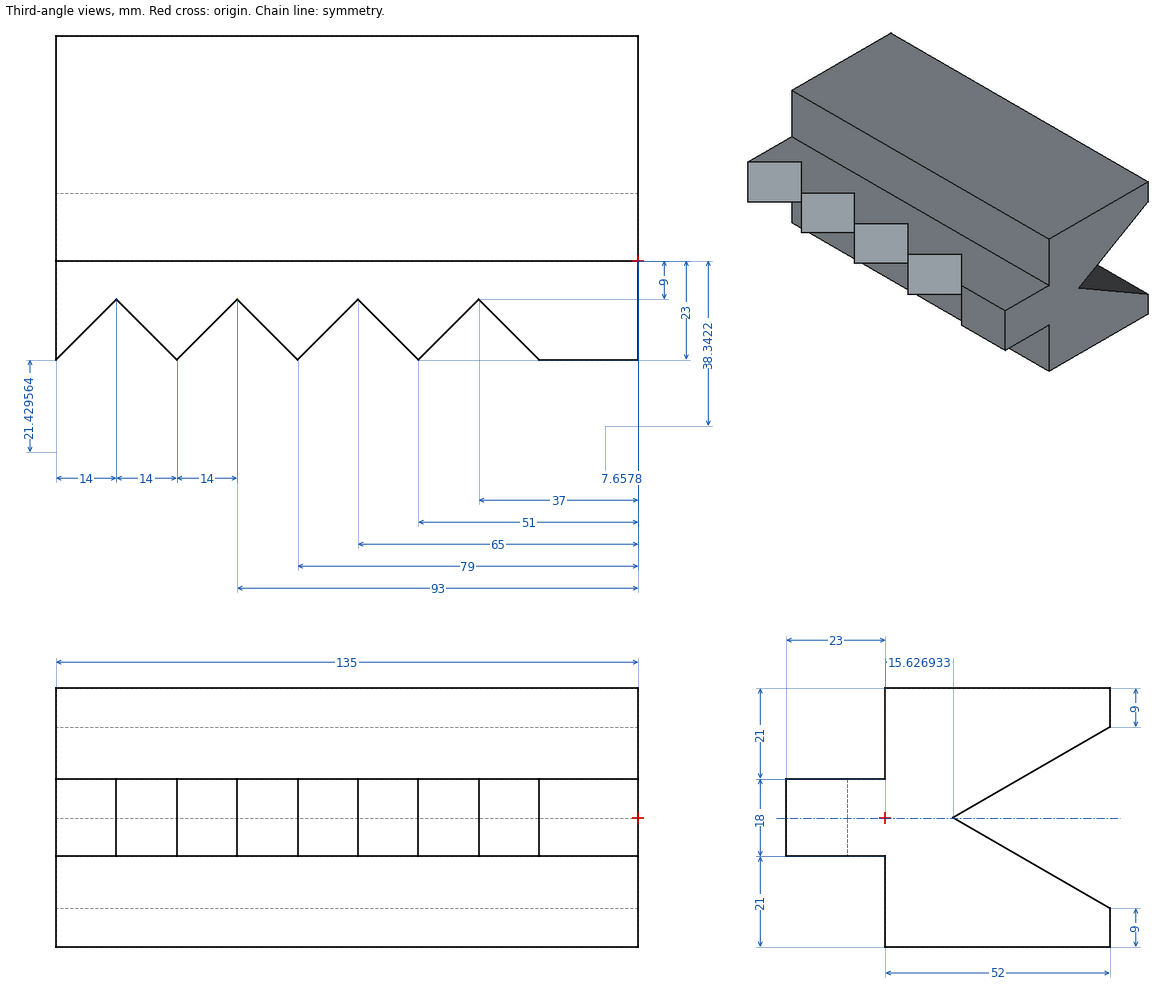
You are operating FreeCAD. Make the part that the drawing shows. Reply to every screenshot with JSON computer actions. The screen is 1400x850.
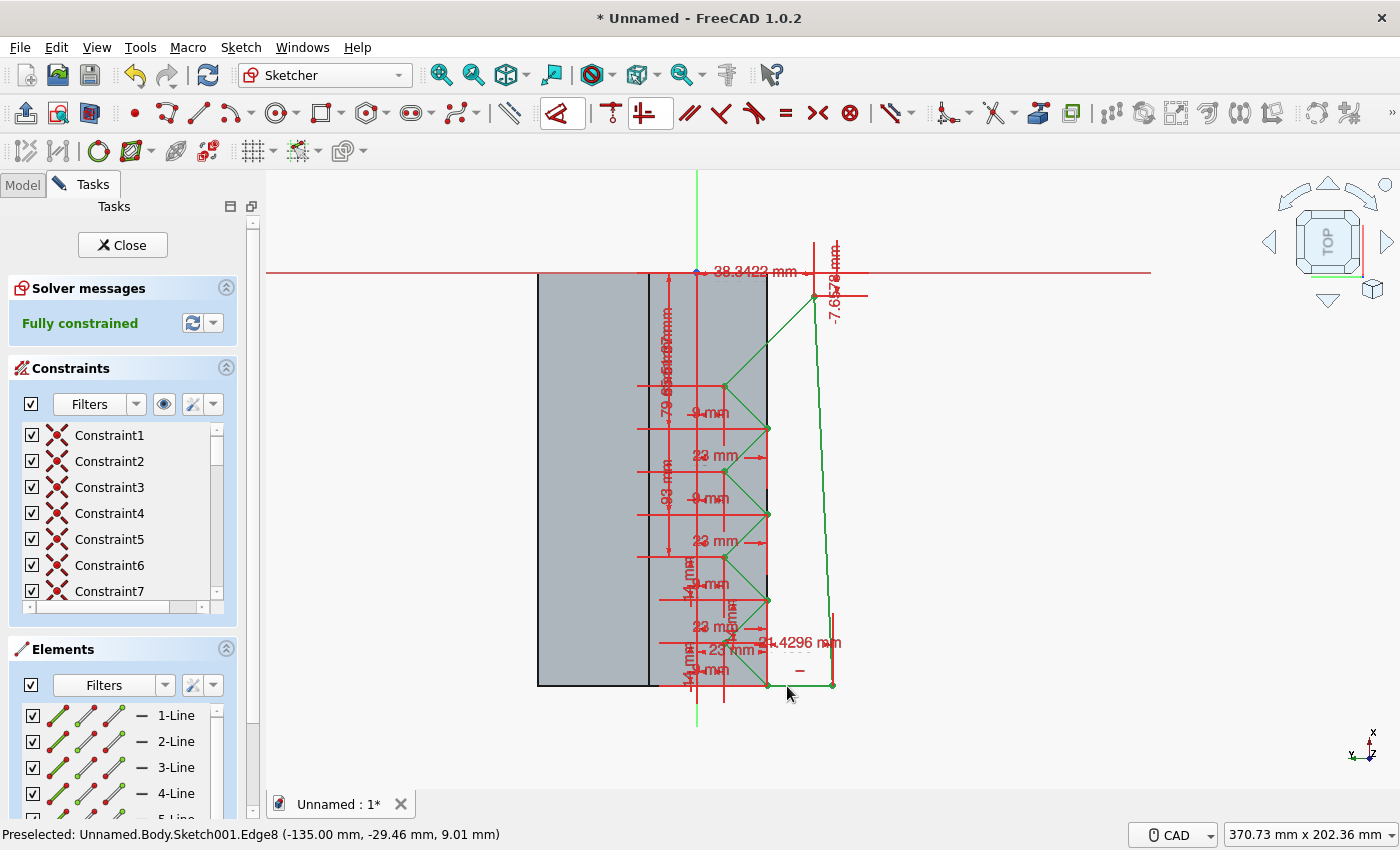
{"action": "left_click", "coordinate": [123, 245]}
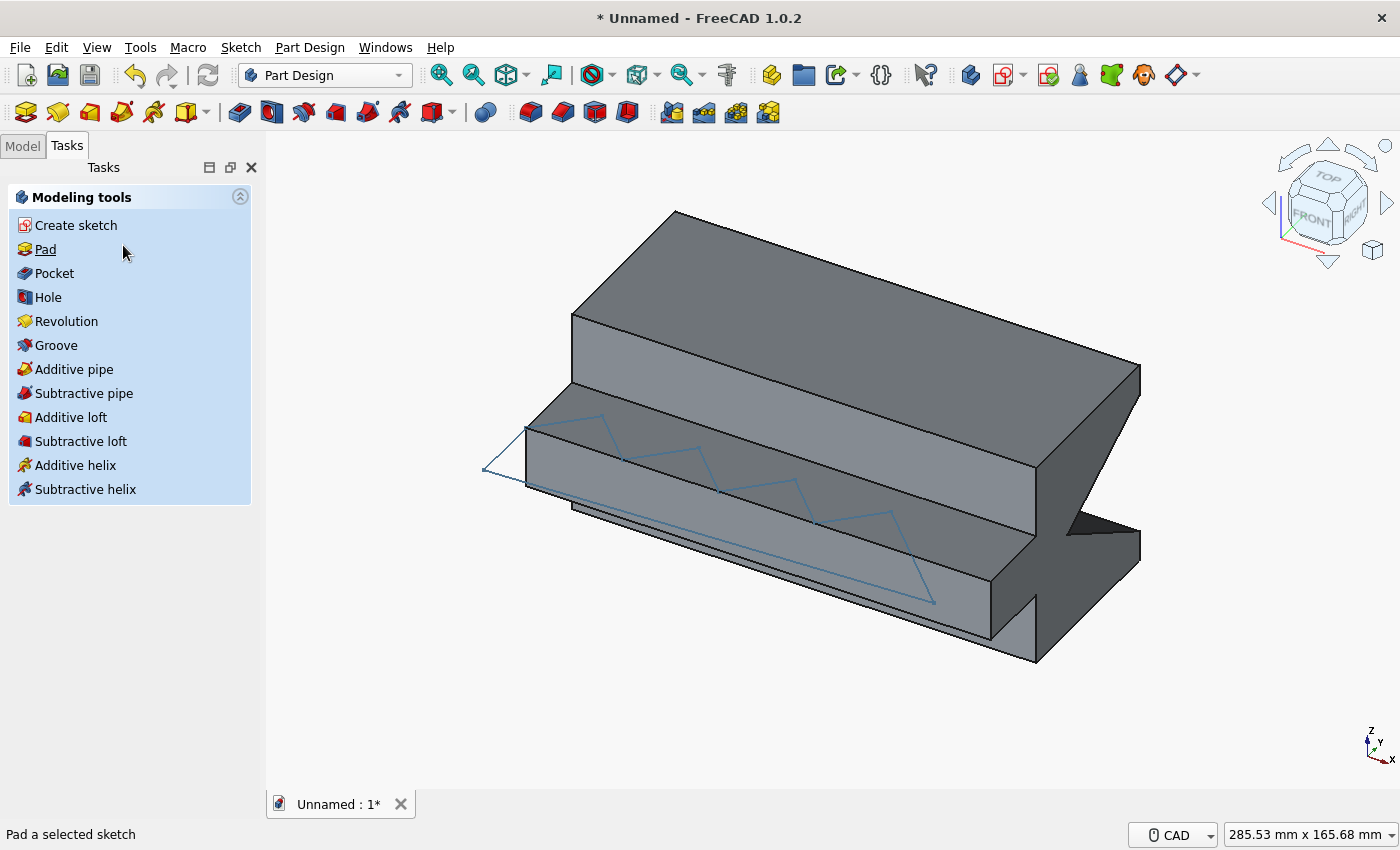
{"action": "left_click", "coordinate": [240, 112]}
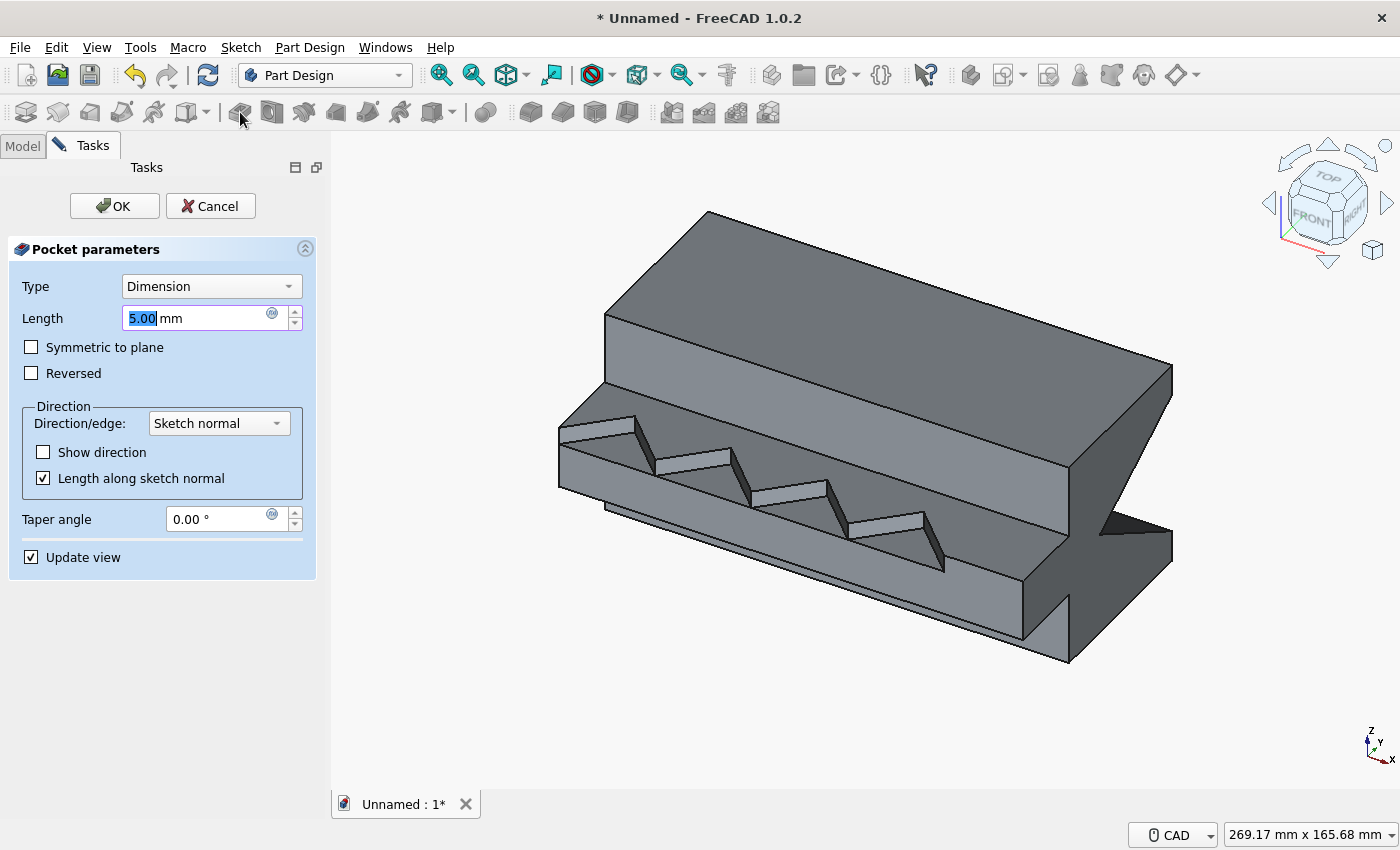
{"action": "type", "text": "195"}
{"action": "key", "text": "Tab"}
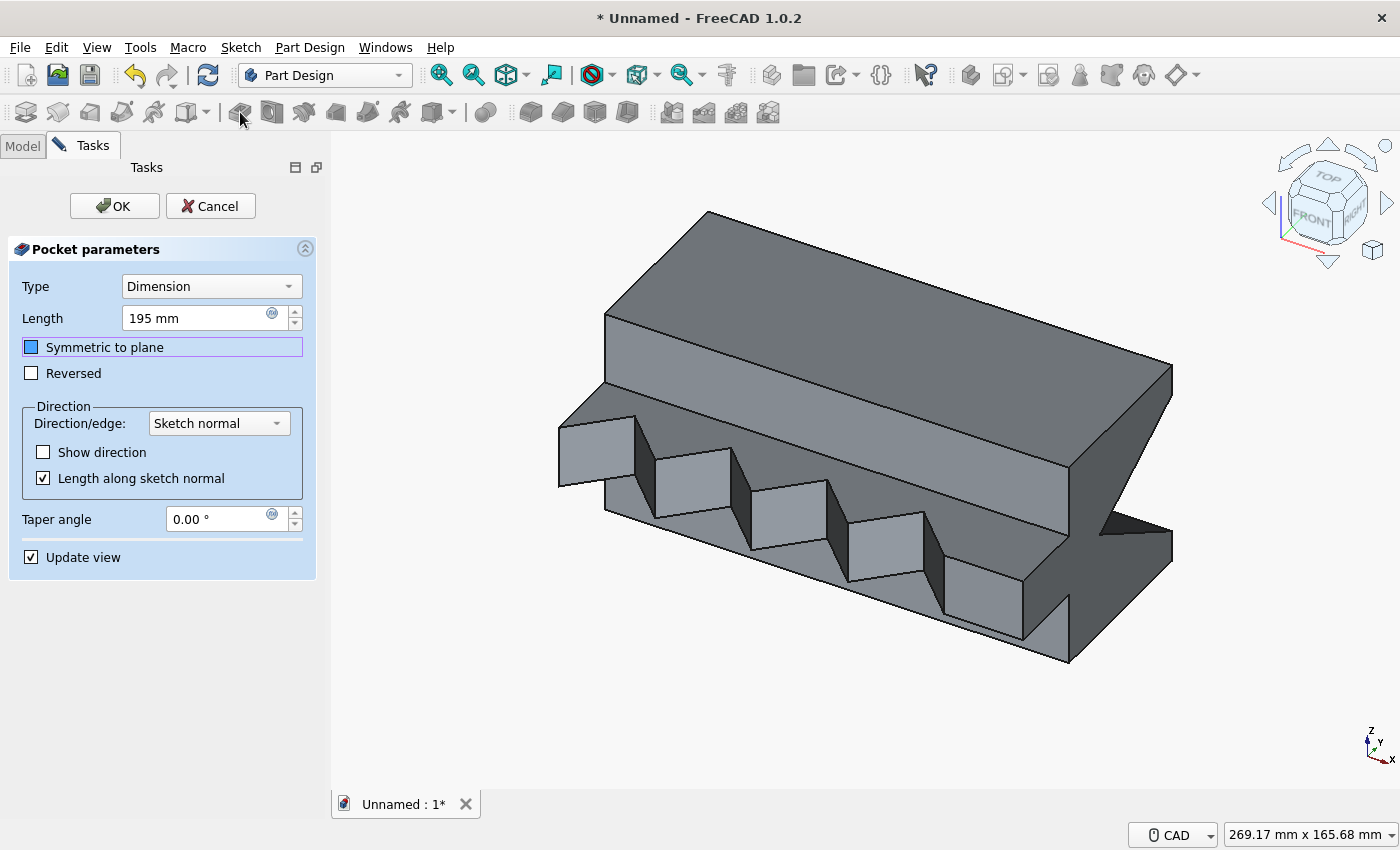
{"action": "left_click", "coordinate": [115, 206]}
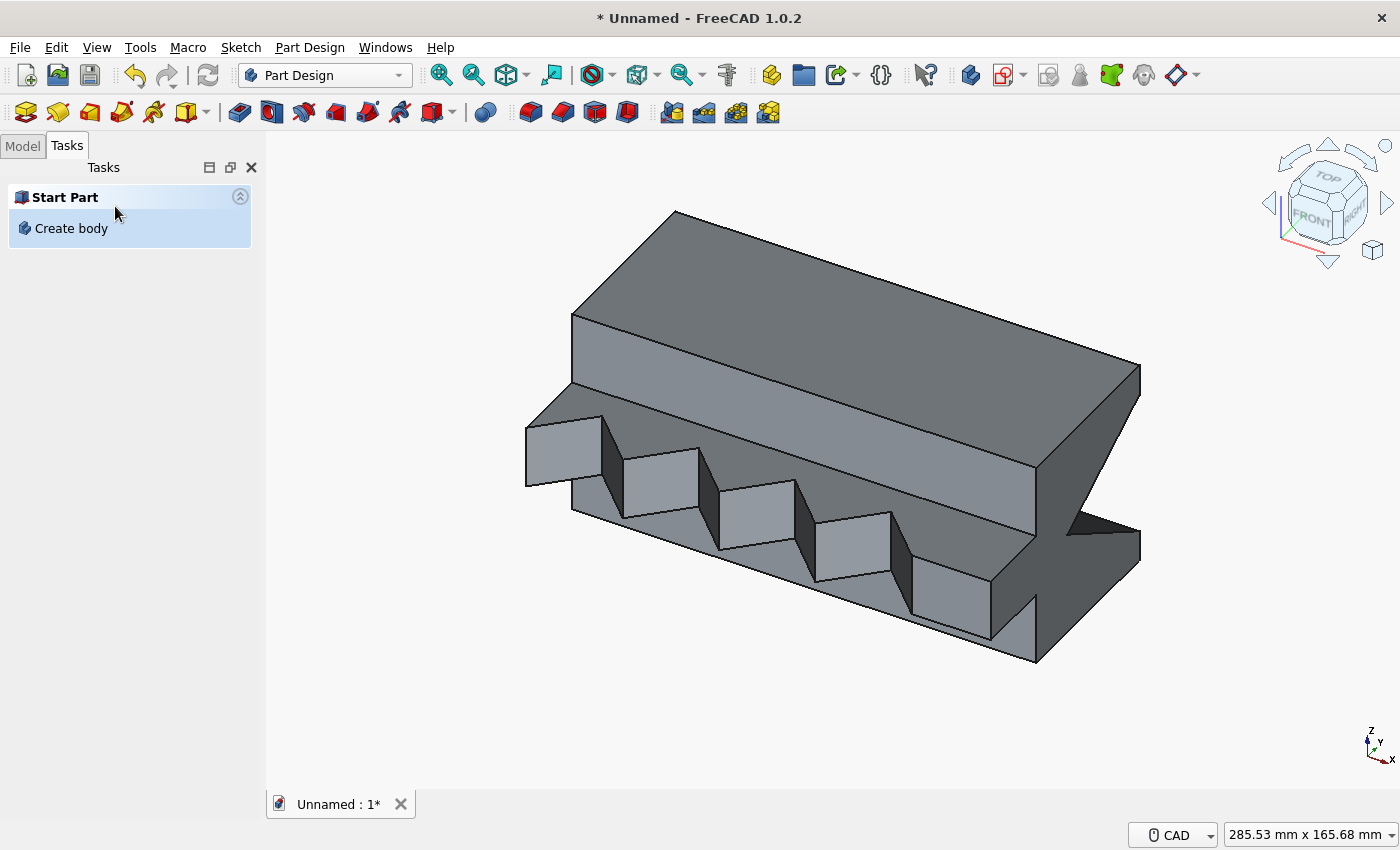
{"action": "key", "text": "0"}